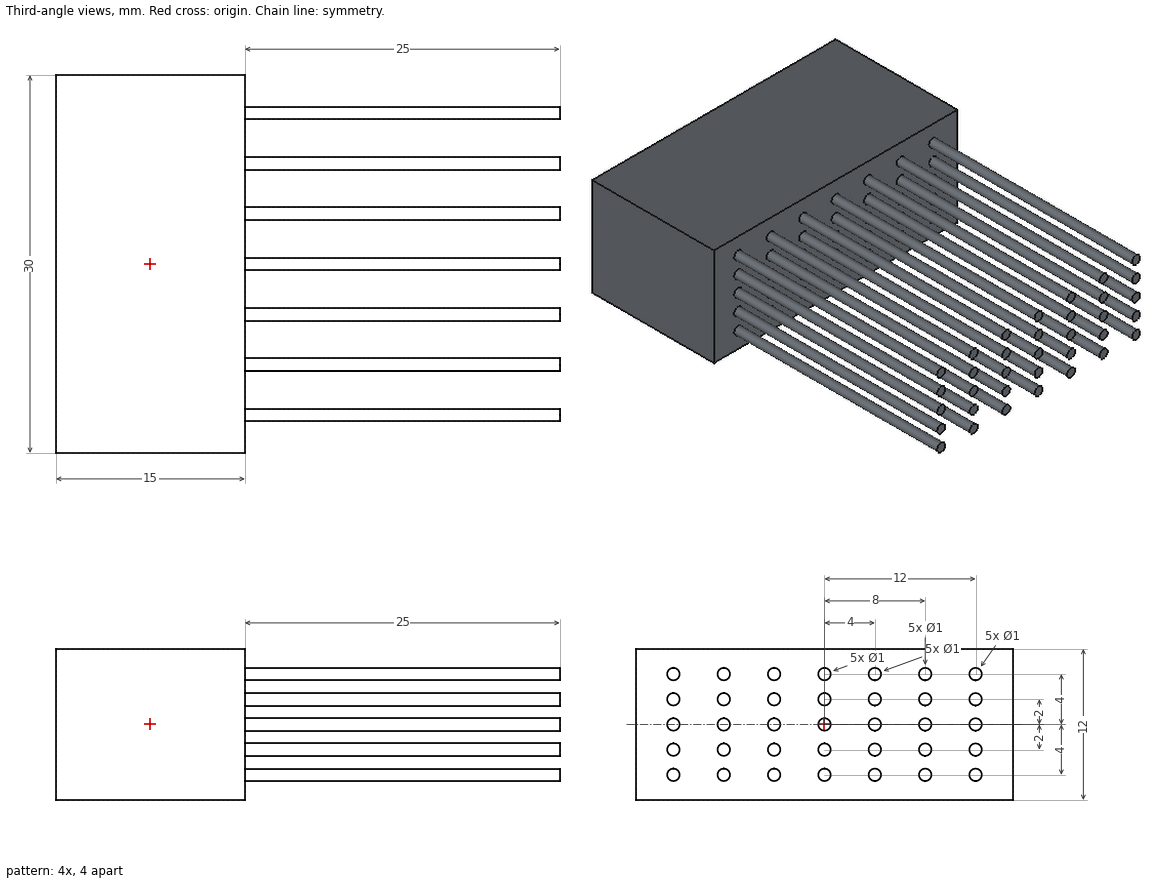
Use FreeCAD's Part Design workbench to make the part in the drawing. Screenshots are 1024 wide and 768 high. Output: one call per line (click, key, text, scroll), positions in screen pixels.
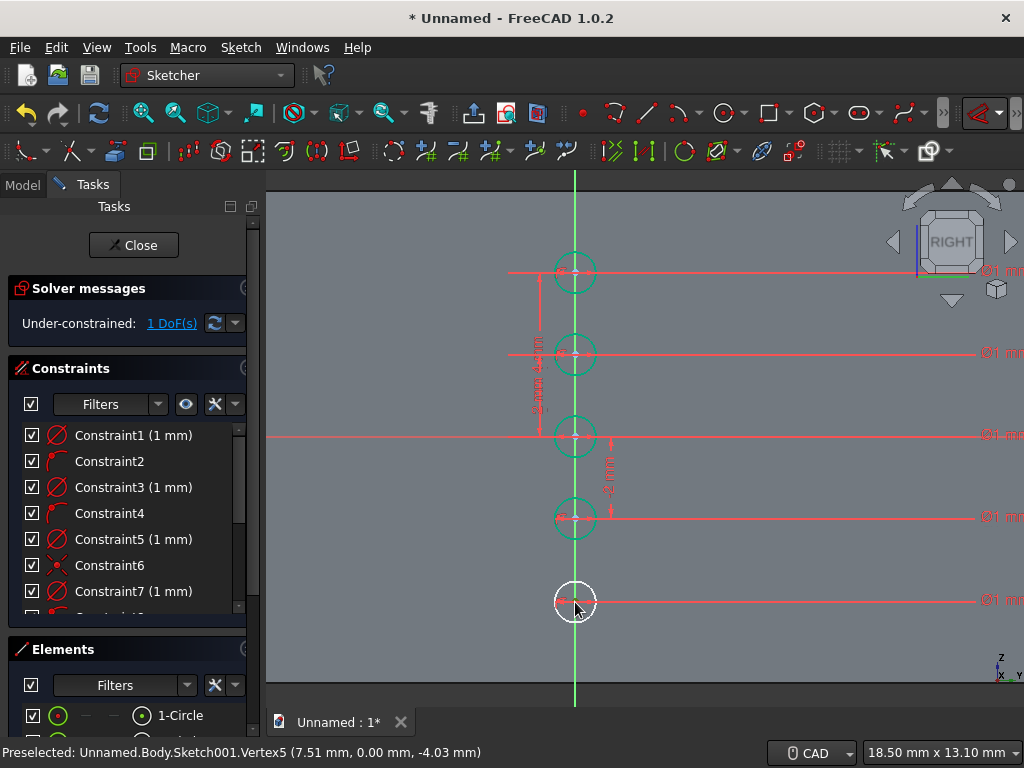
key(i)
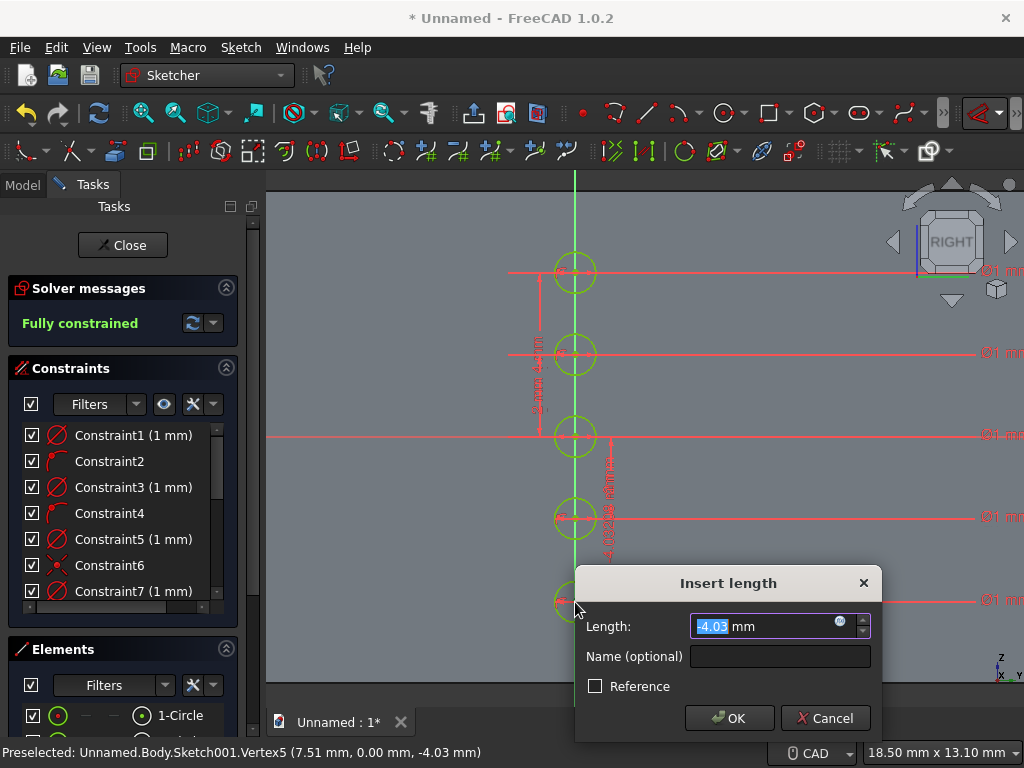
text(-4)
key(Return)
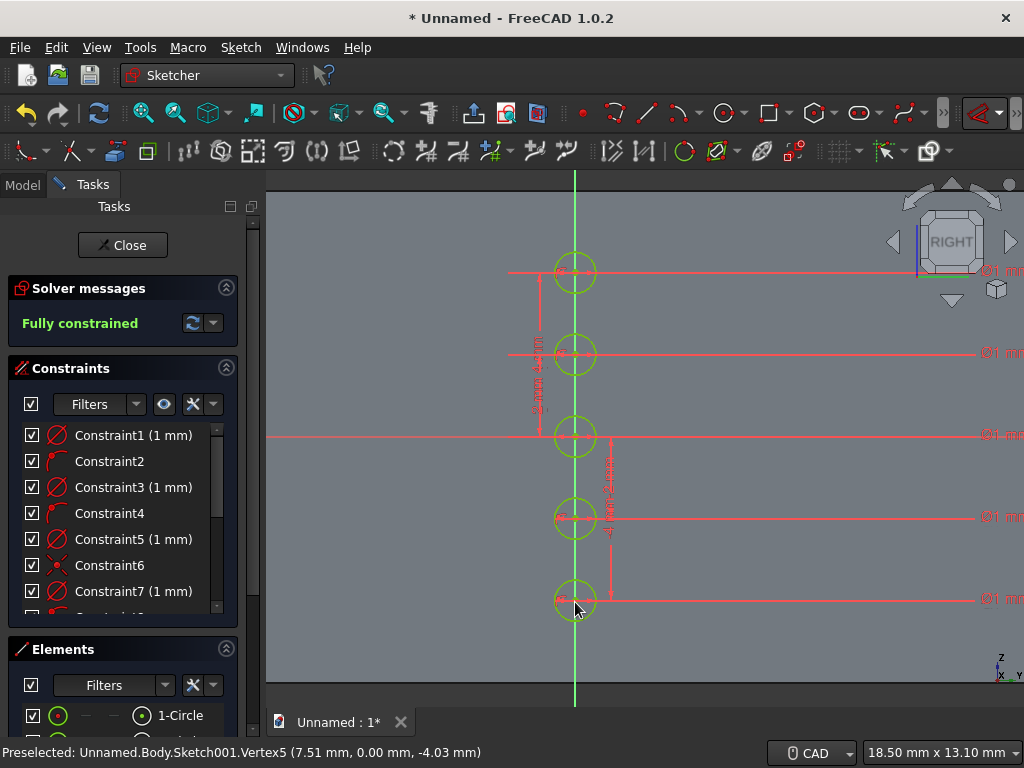
click(123, 245)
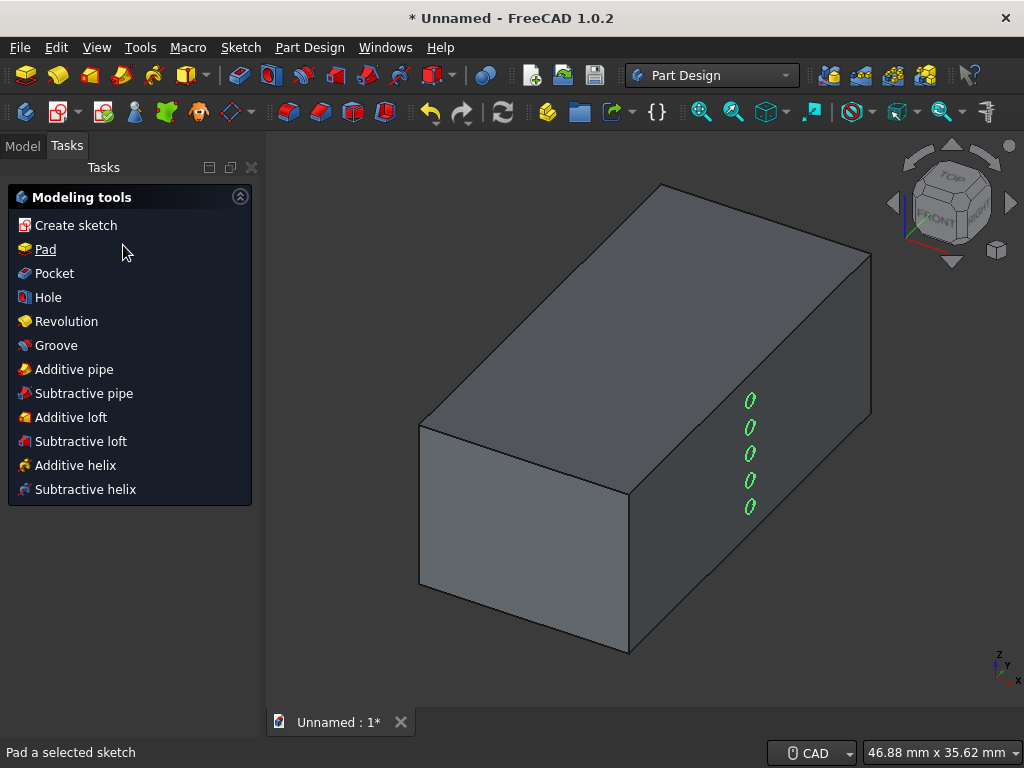
click(26, 76)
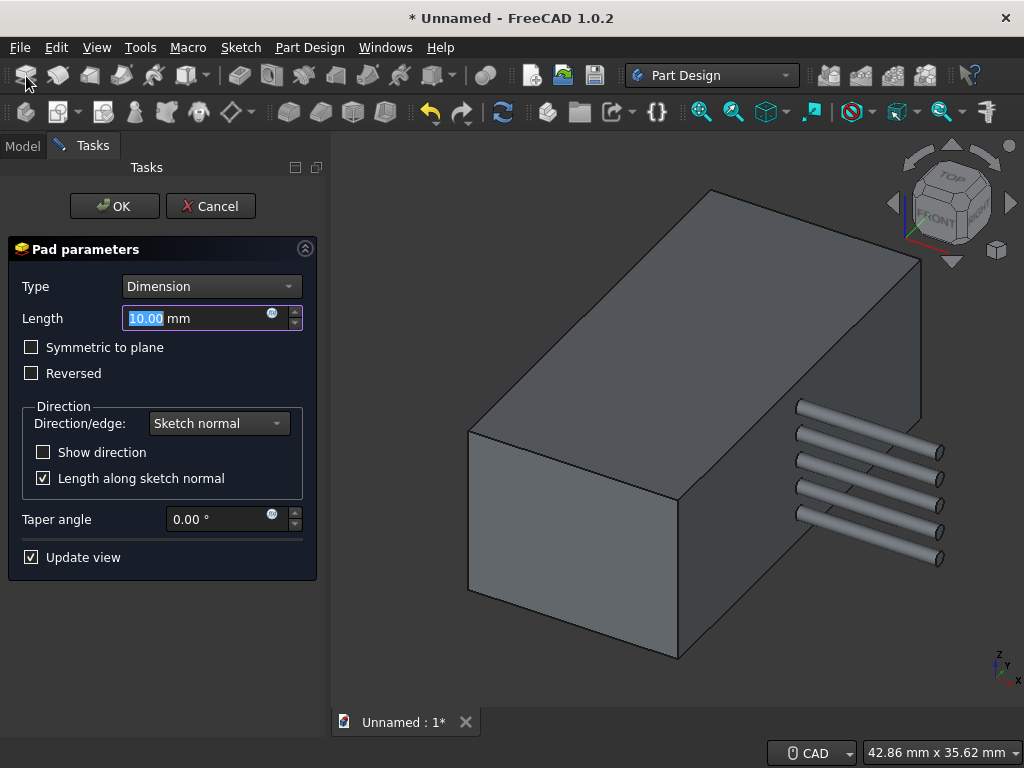
text(25)
key(Tab)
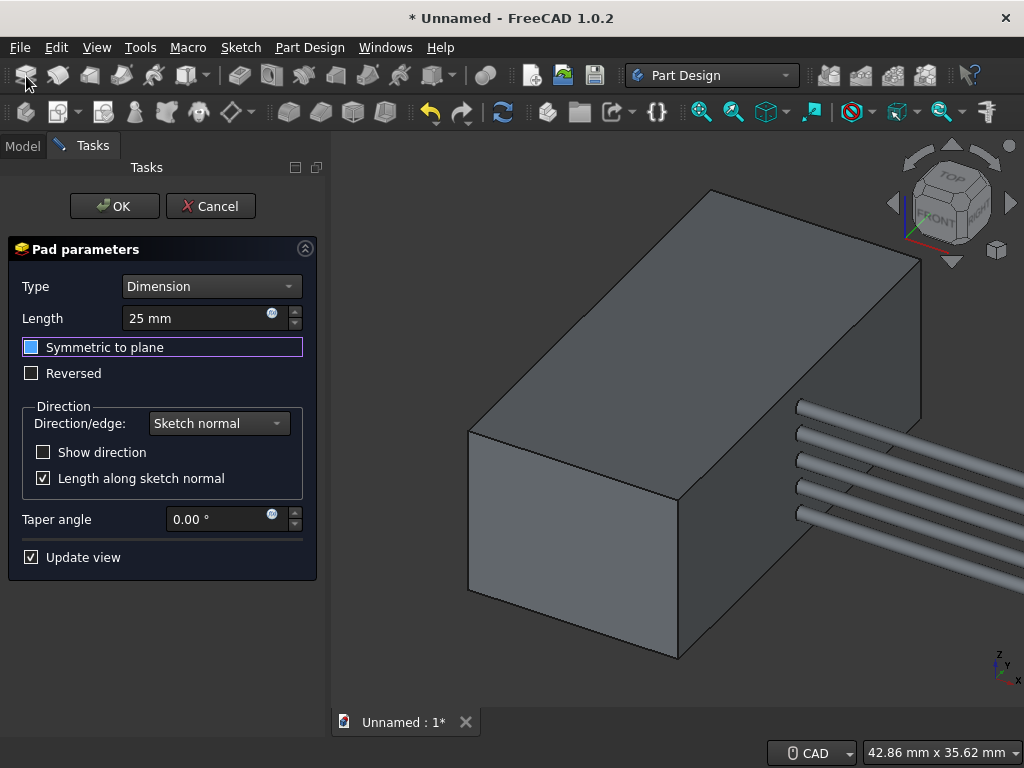
click(115, 206)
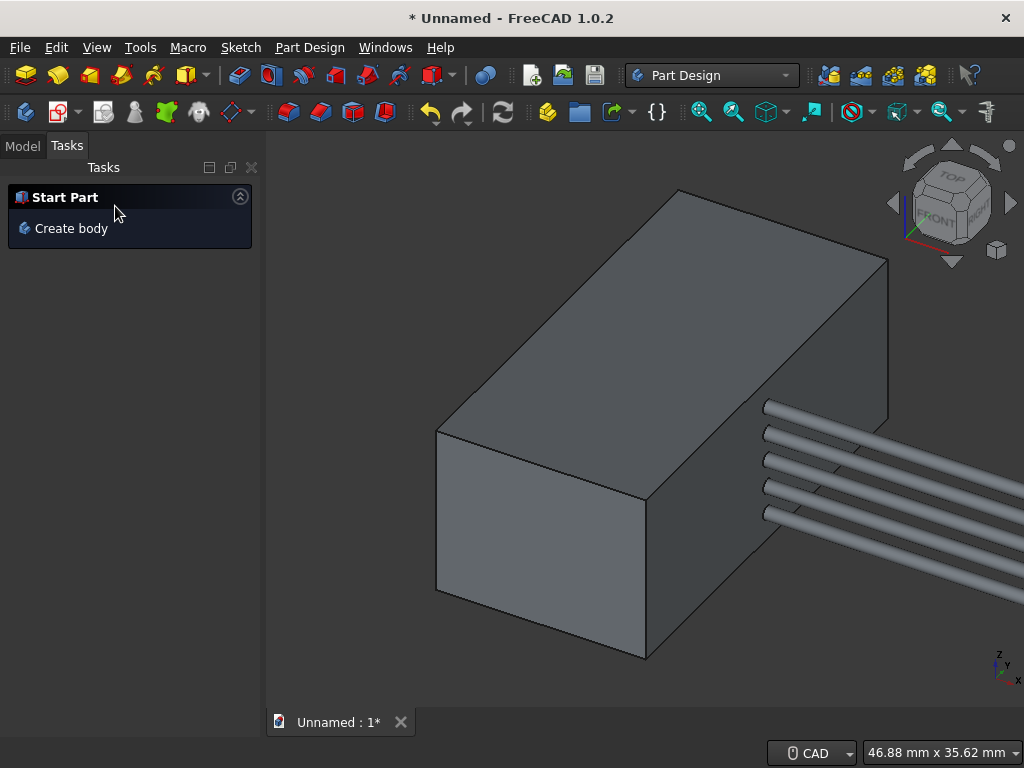
key(v)
key(f)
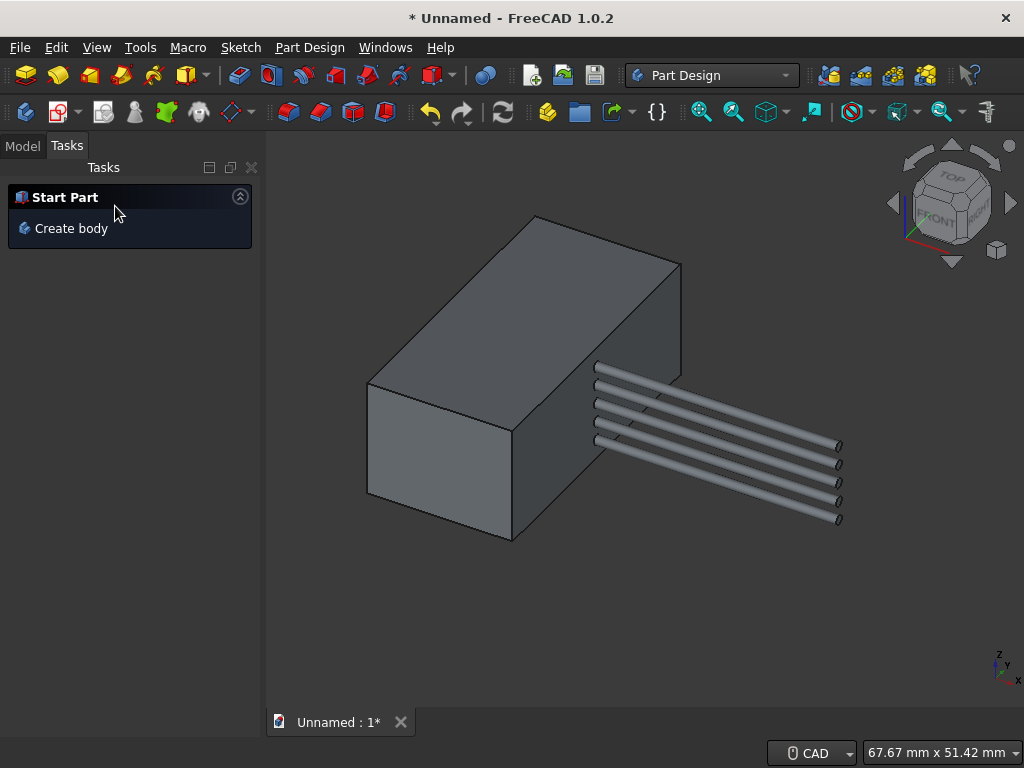
click(23, 145)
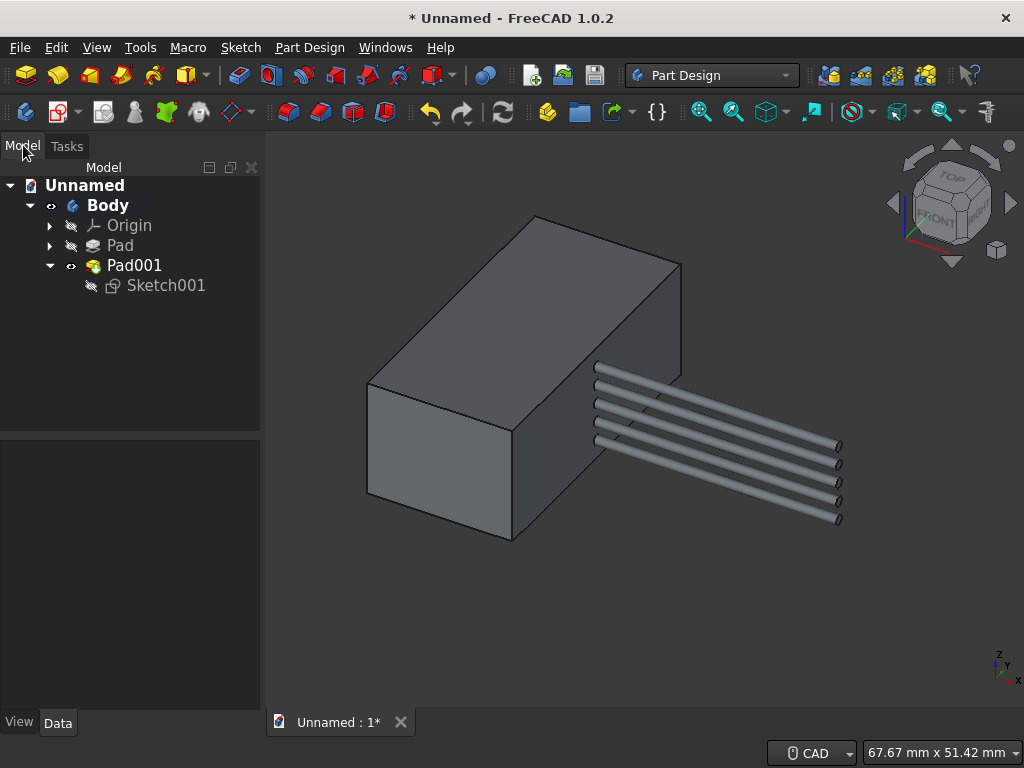
click(116, 266)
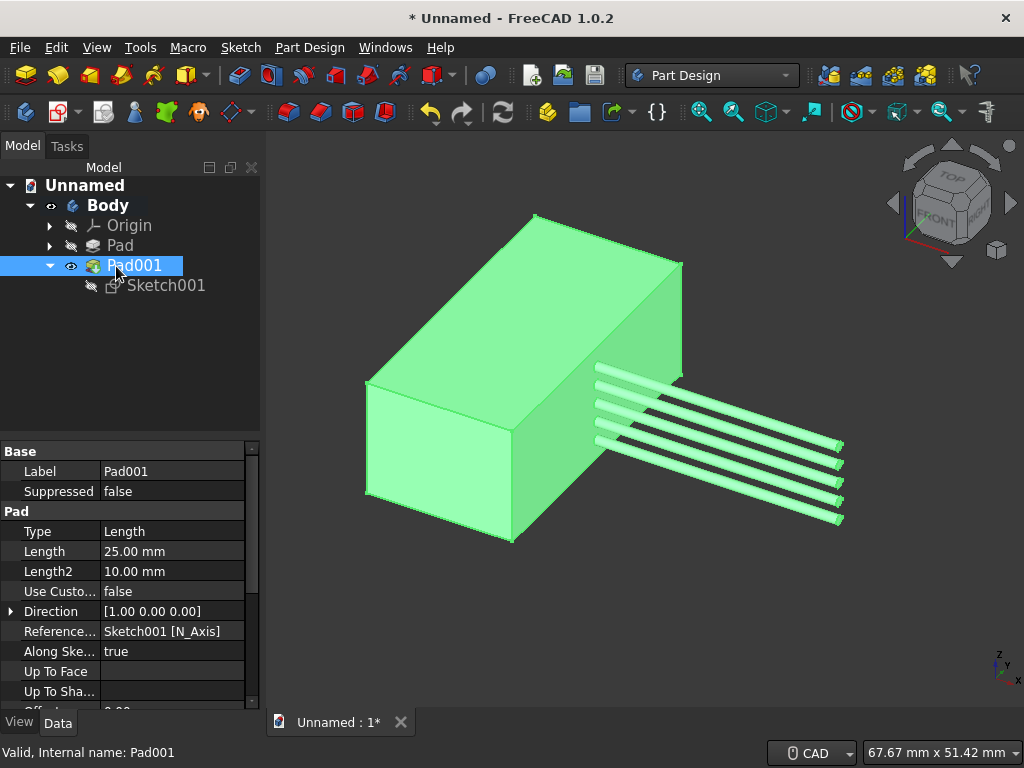
click(862, 76)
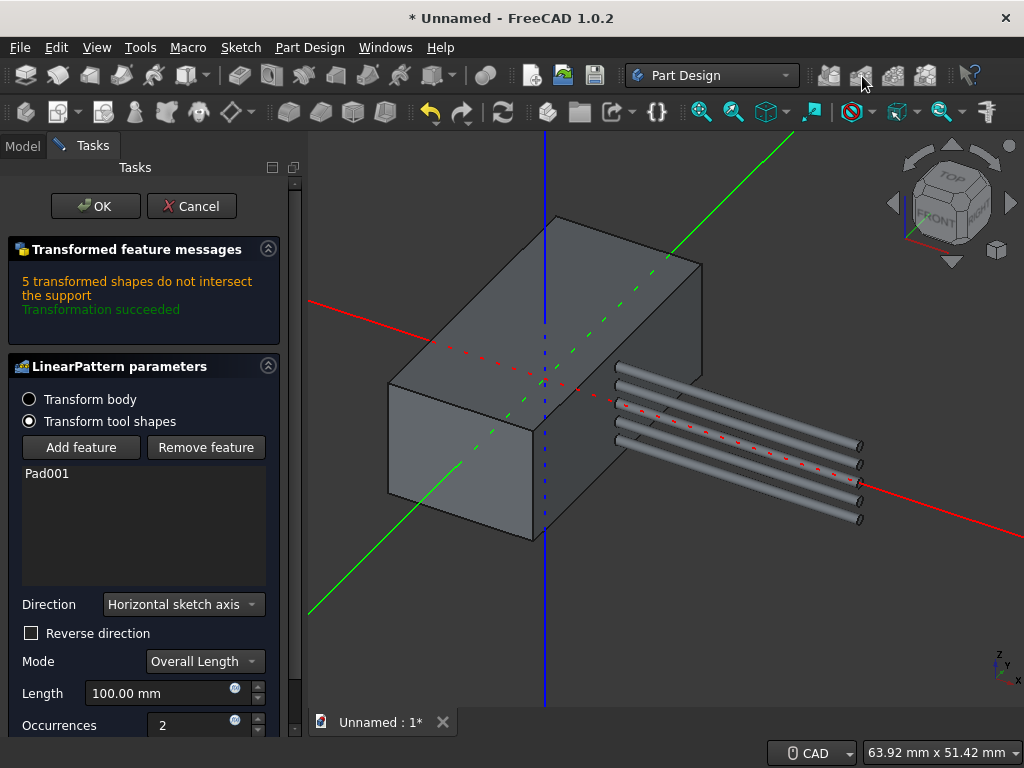
click(184, 604)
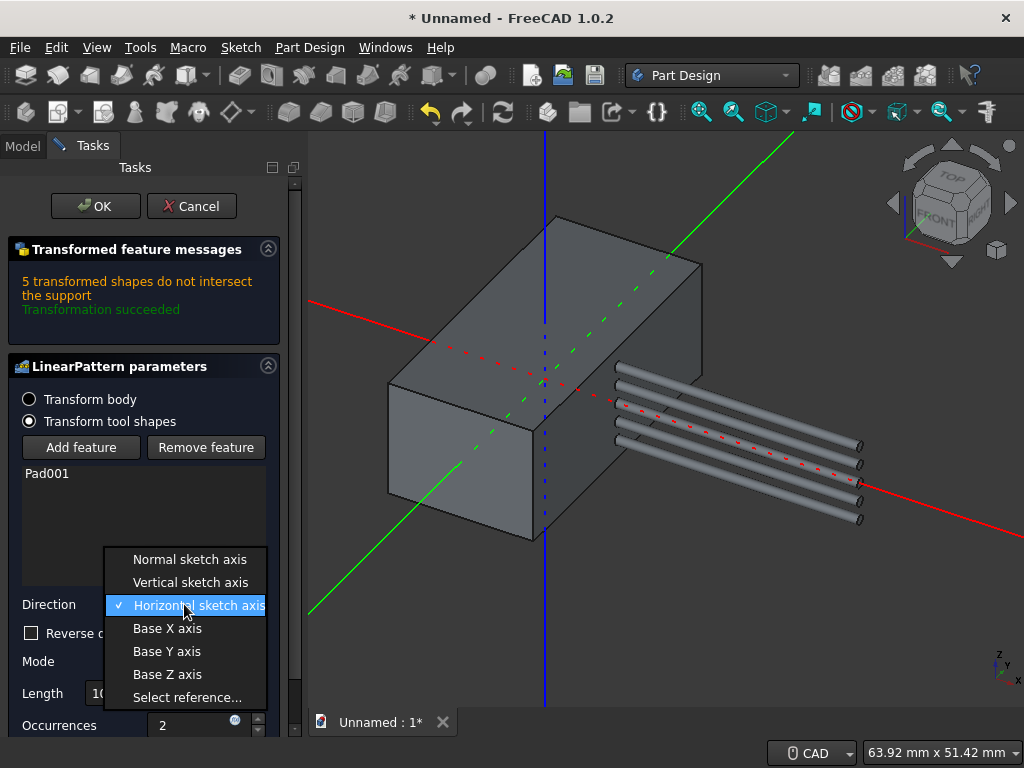
click(184, 652)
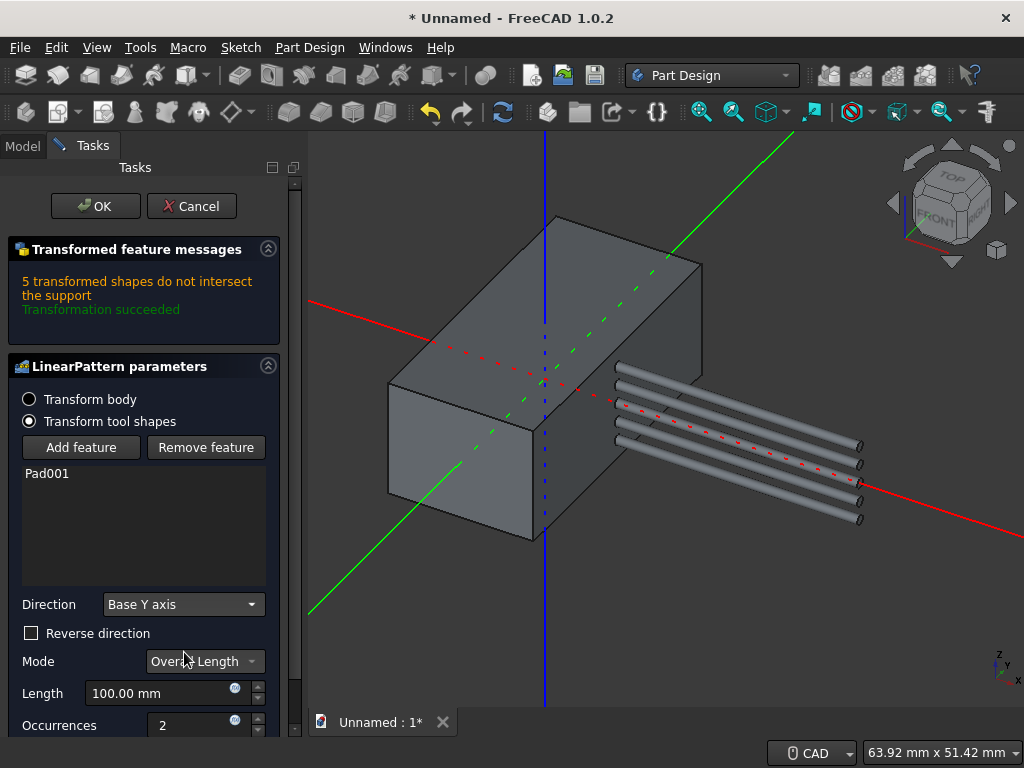
click(206, 662)